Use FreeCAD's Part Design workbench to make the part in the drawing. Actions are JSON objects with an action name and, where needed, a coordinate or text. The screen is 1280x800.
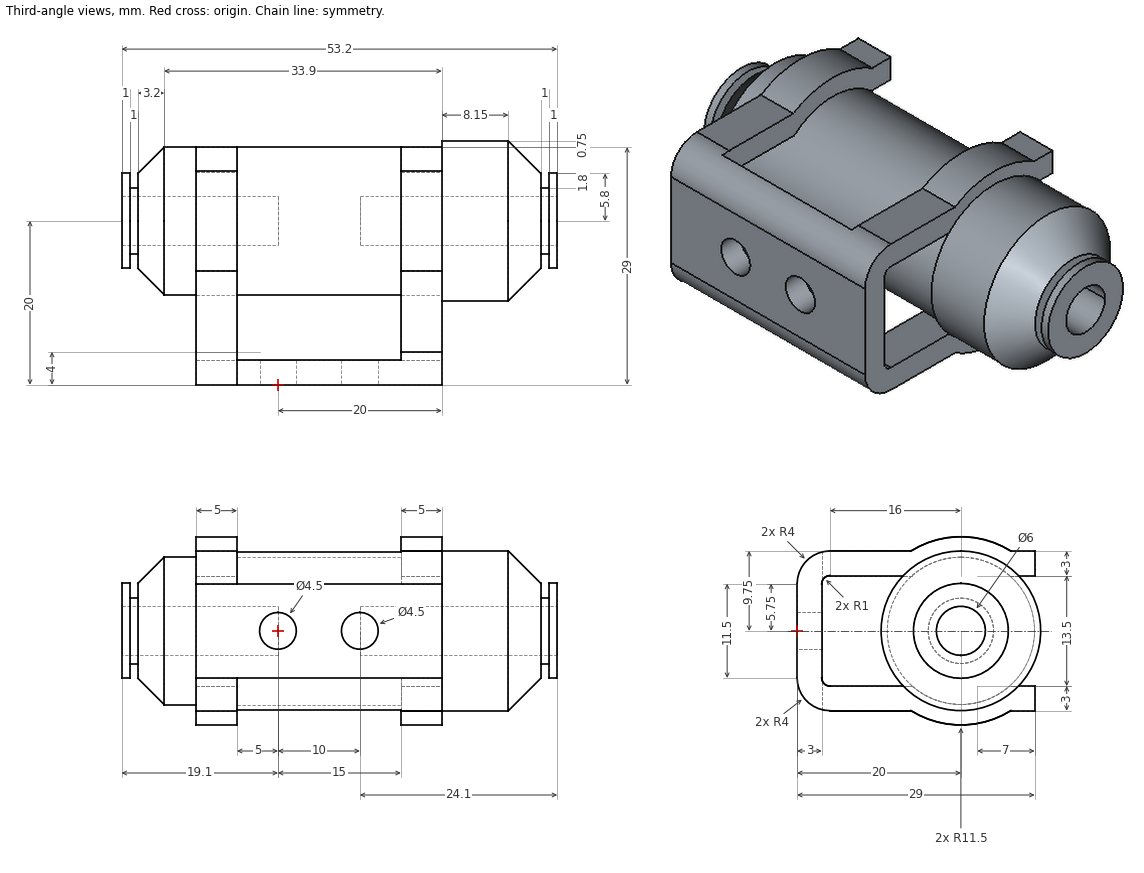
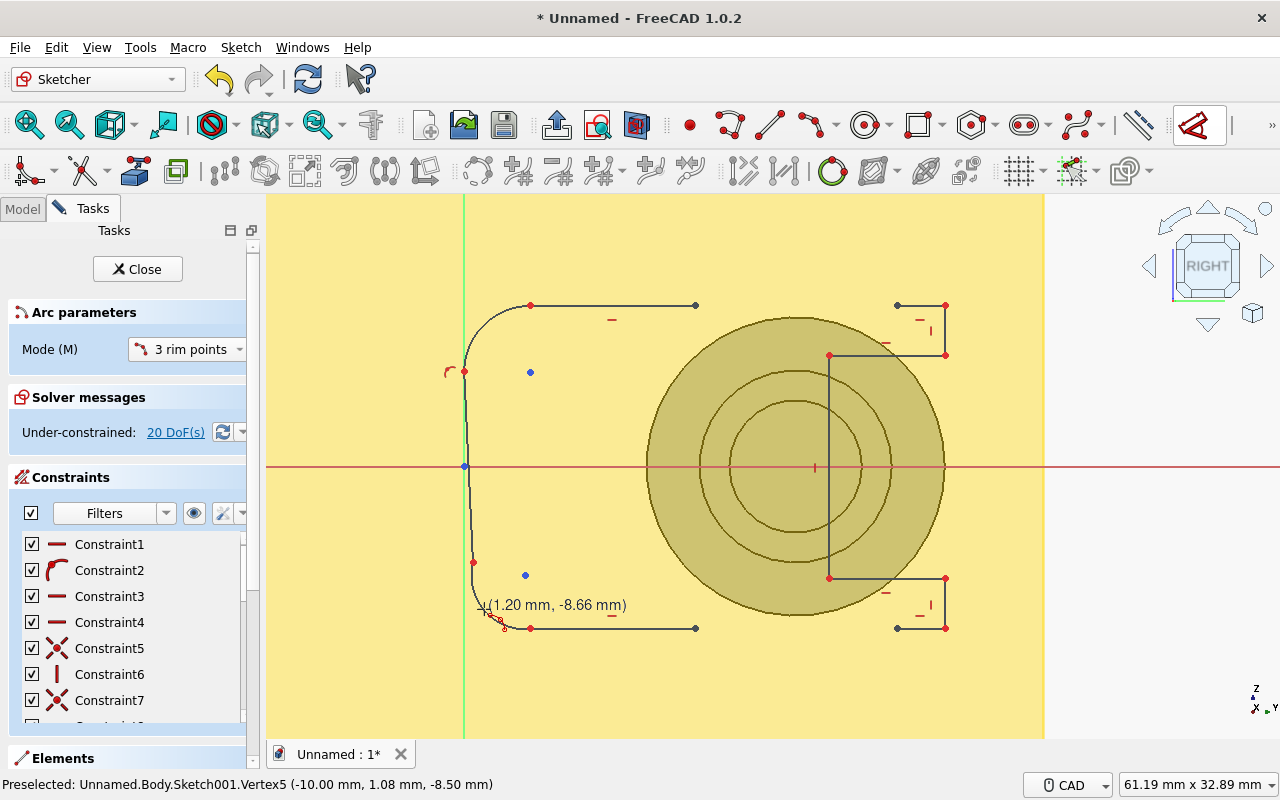
{"action": "left_click", "coordinate": [695, 629]}
{"action": "left_click", "coordinate": [897, 629]}
{"action": "left_click", "coordinate": [796, 657]}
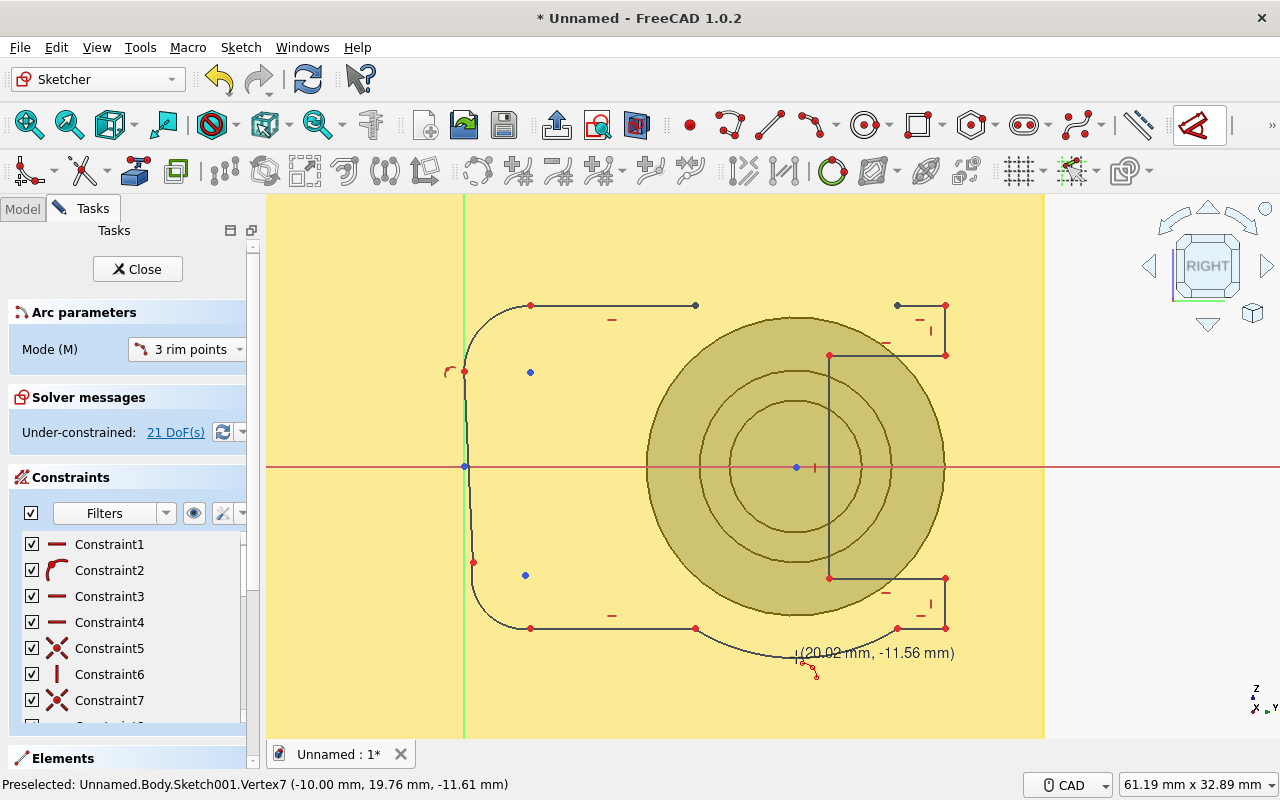
{"action": "left_click", "coordinate": [897, 306]}
{"action": "left_click", "coordinate": [695, 306]}
{"action": "left_click", "coordinate": [796, 276]}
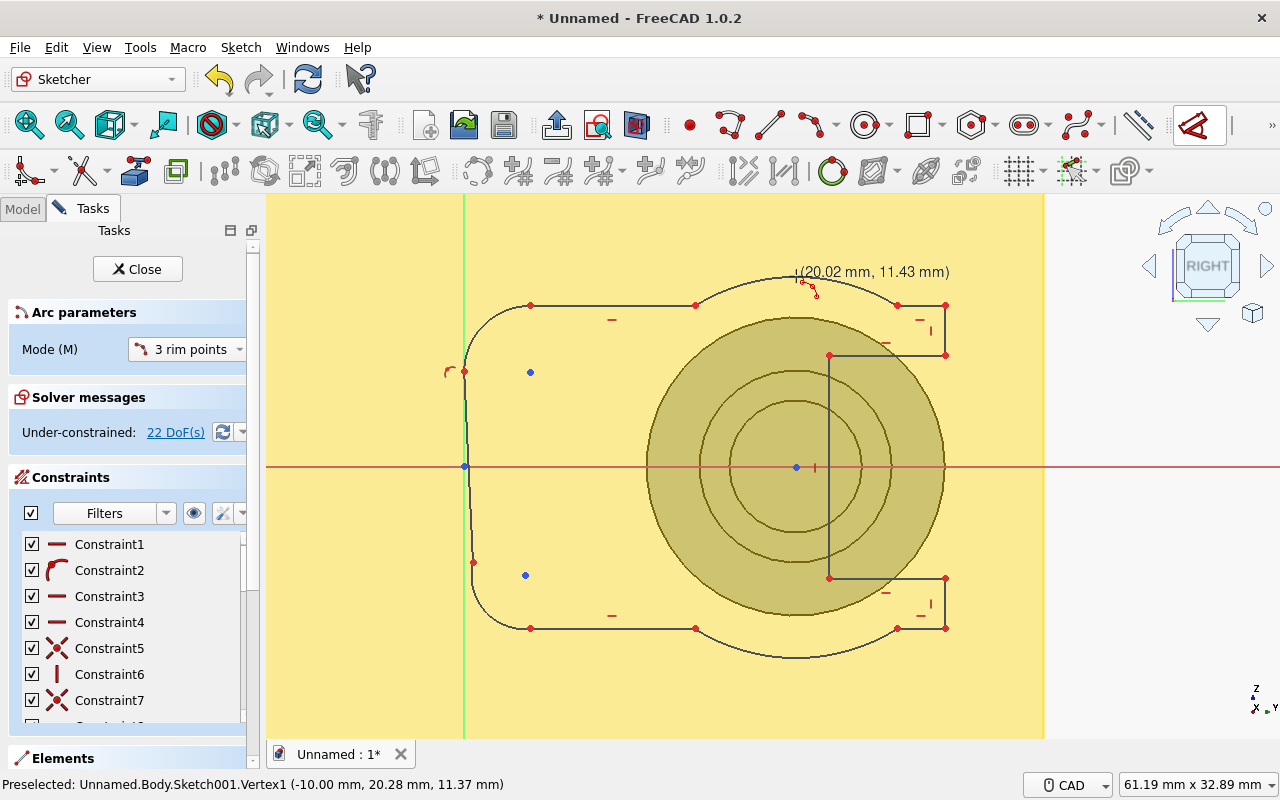
{"action": "left_click", "coordinate": [770, 126]}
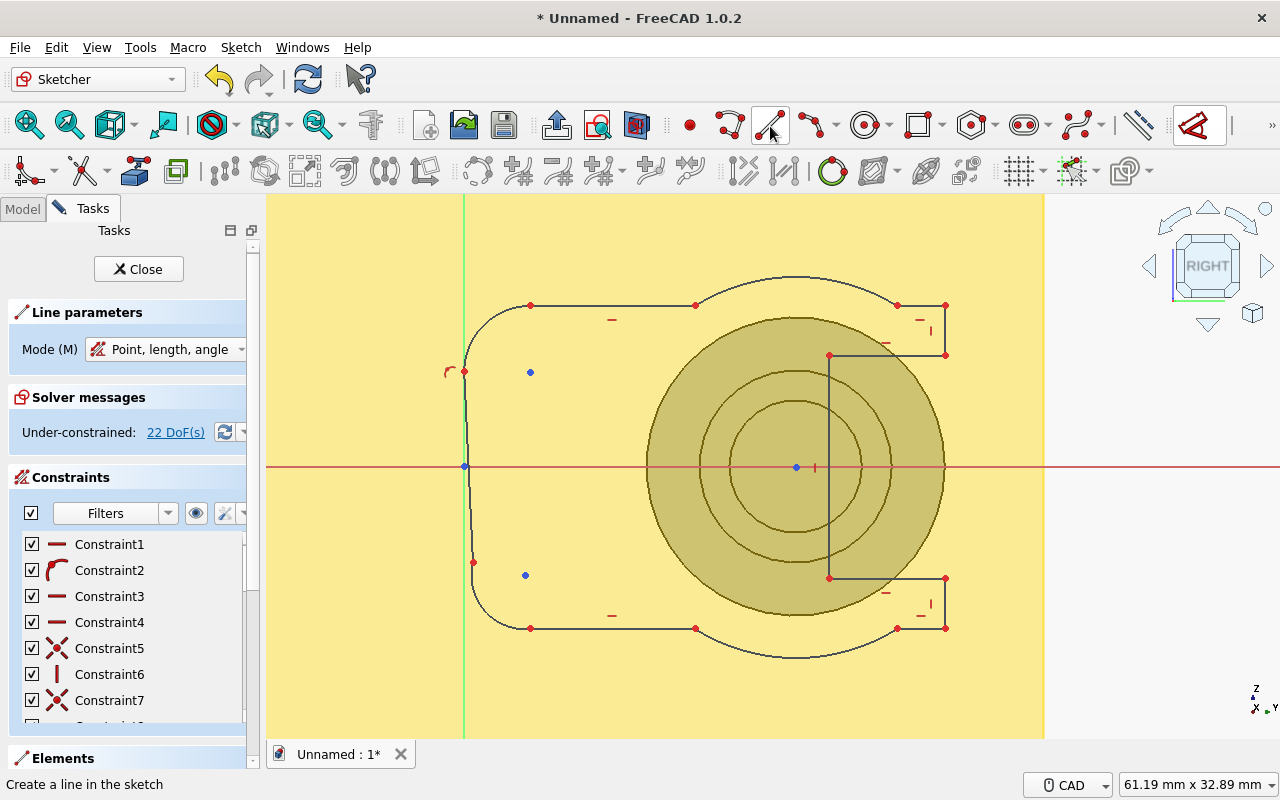
{"action": "left_click", "coordinate": [514, 562]}
{"action": "left_click", "coordinate": [514, 371]}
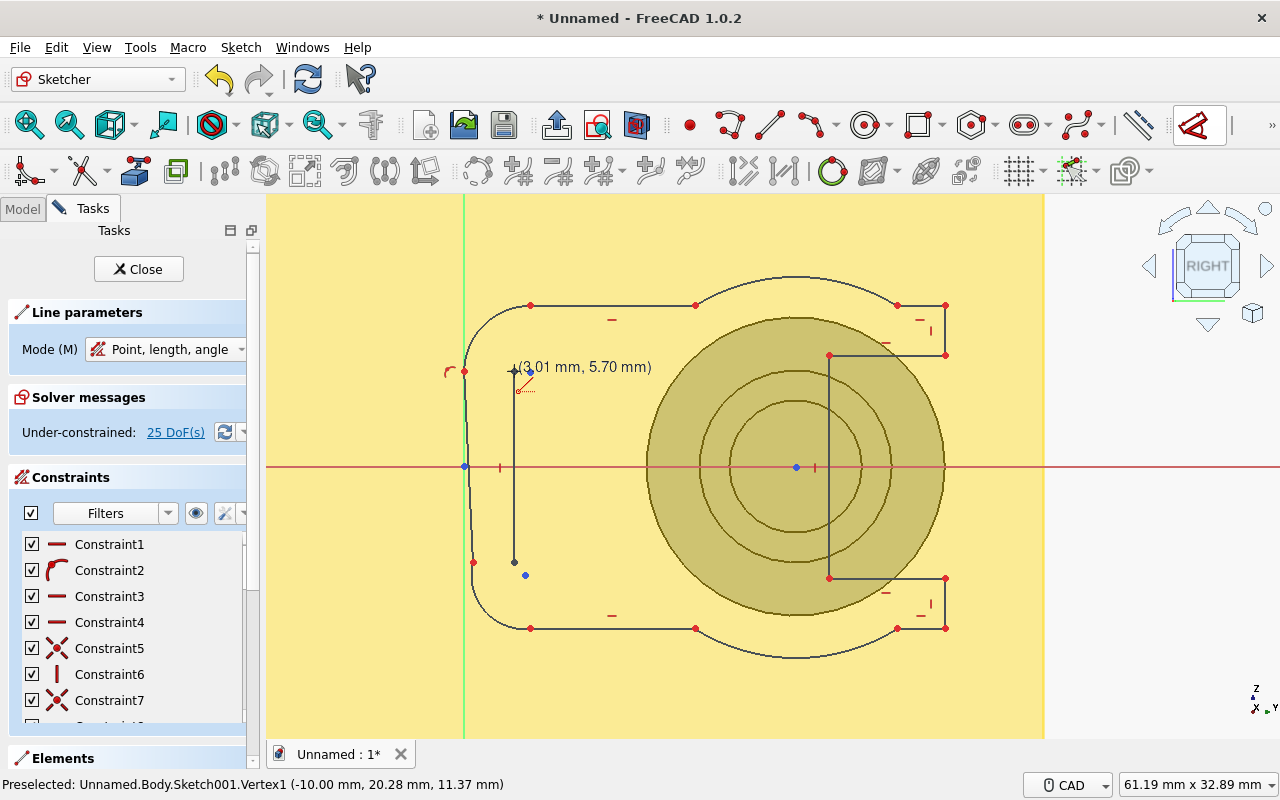
{"action": "left_click", "coordinate": [730, 126]}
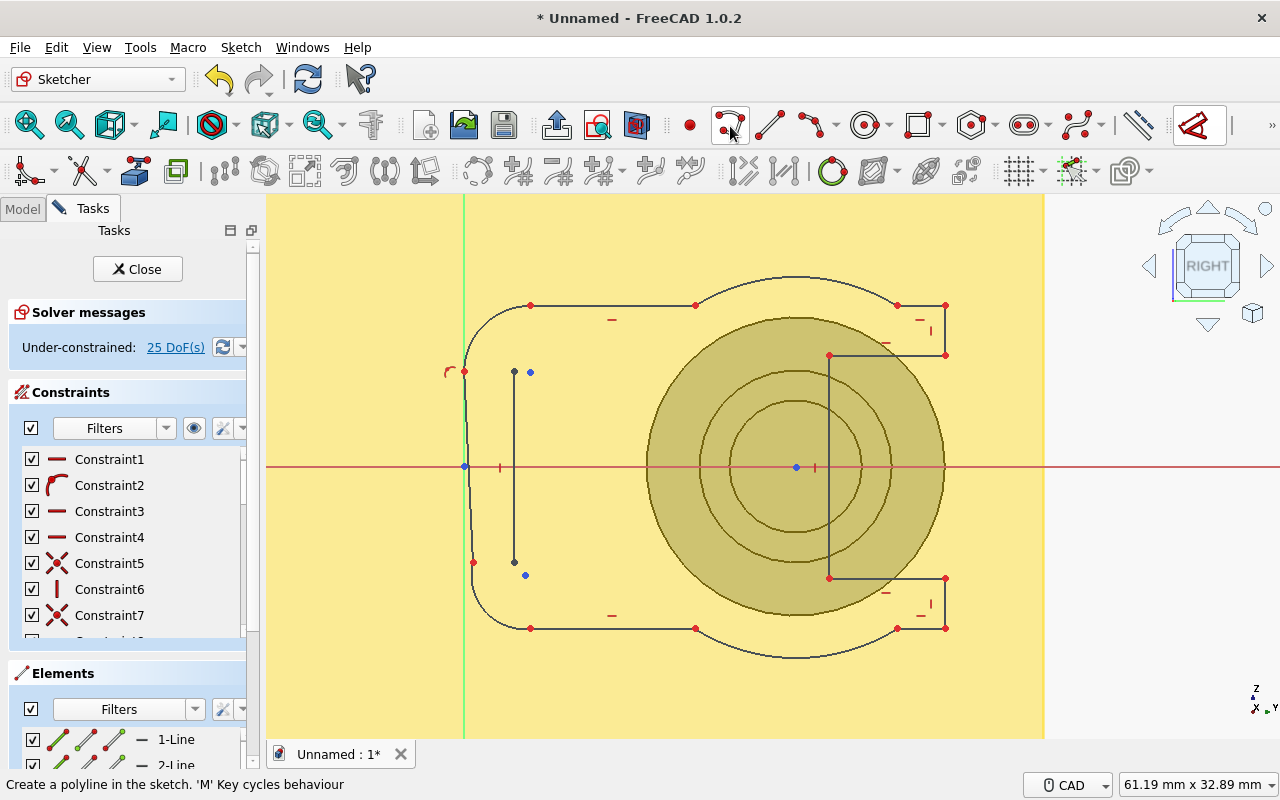
{"action": "left_click", "coordinate": [530, 355]}
{"action": "left_click", "coordinate": [796, 355]}
{"action": "left_click", "coordinate": [796, 578]}
{"action": "left_click", "coordinate": [530, 578]}
{"action": "right_click", "coordinate": [530, 578]}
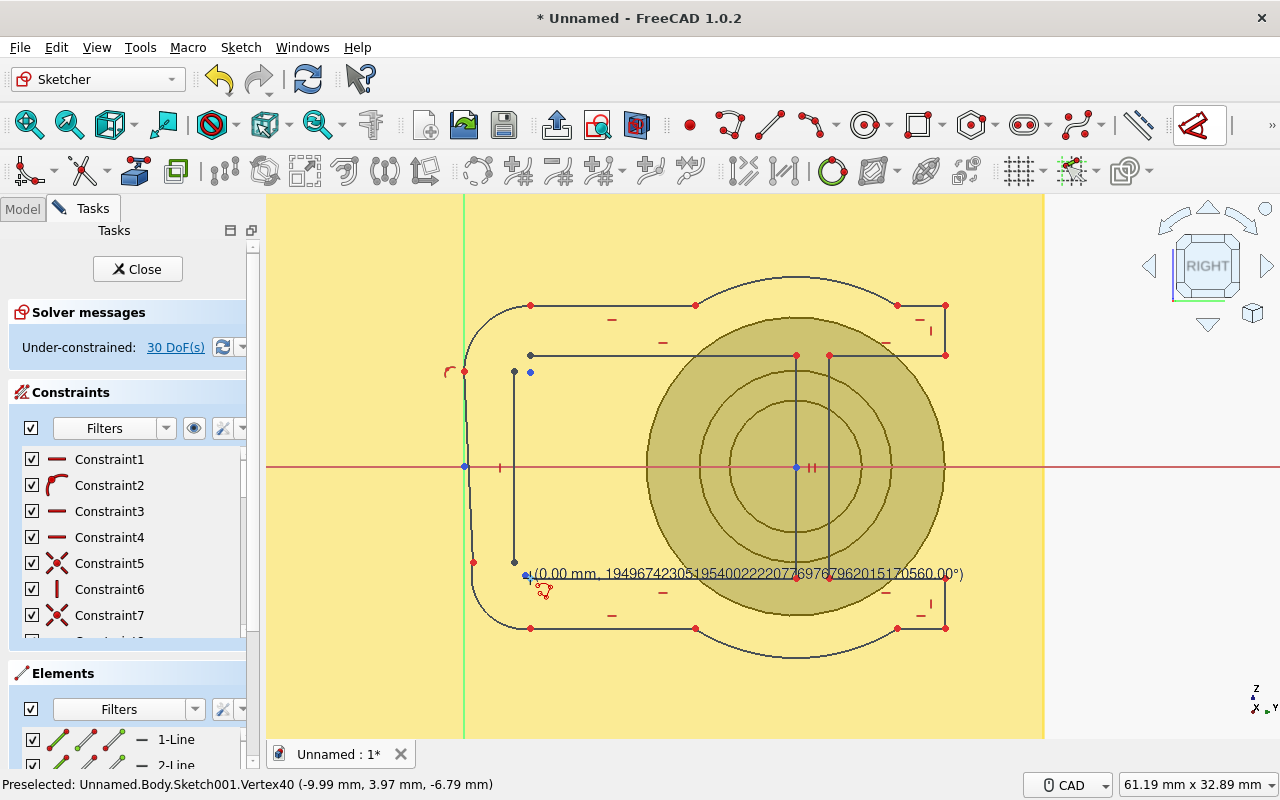
{"action": "left_click", "coordinate": [812, 126]}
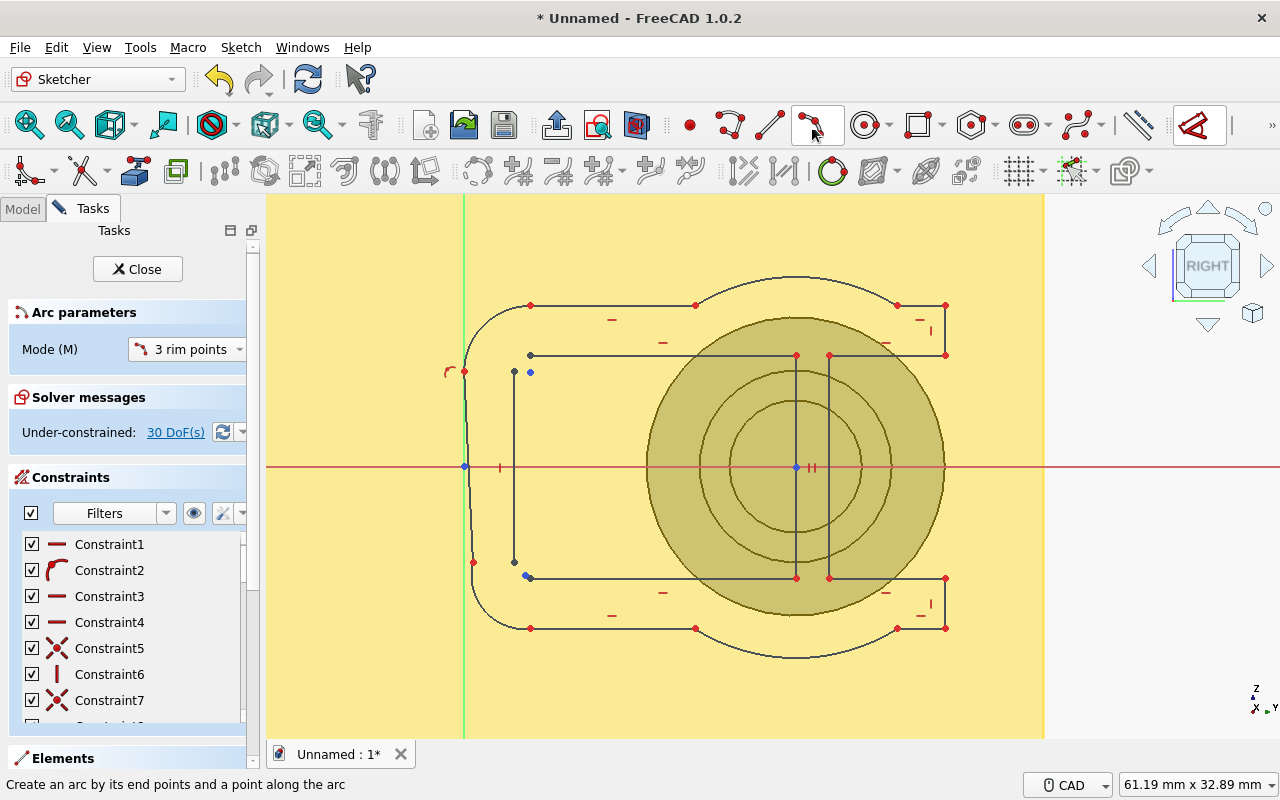
{"action": "left_click", "coordinate": [514, 372]}
{"action": "left_click", "coordinate": [530, 356]}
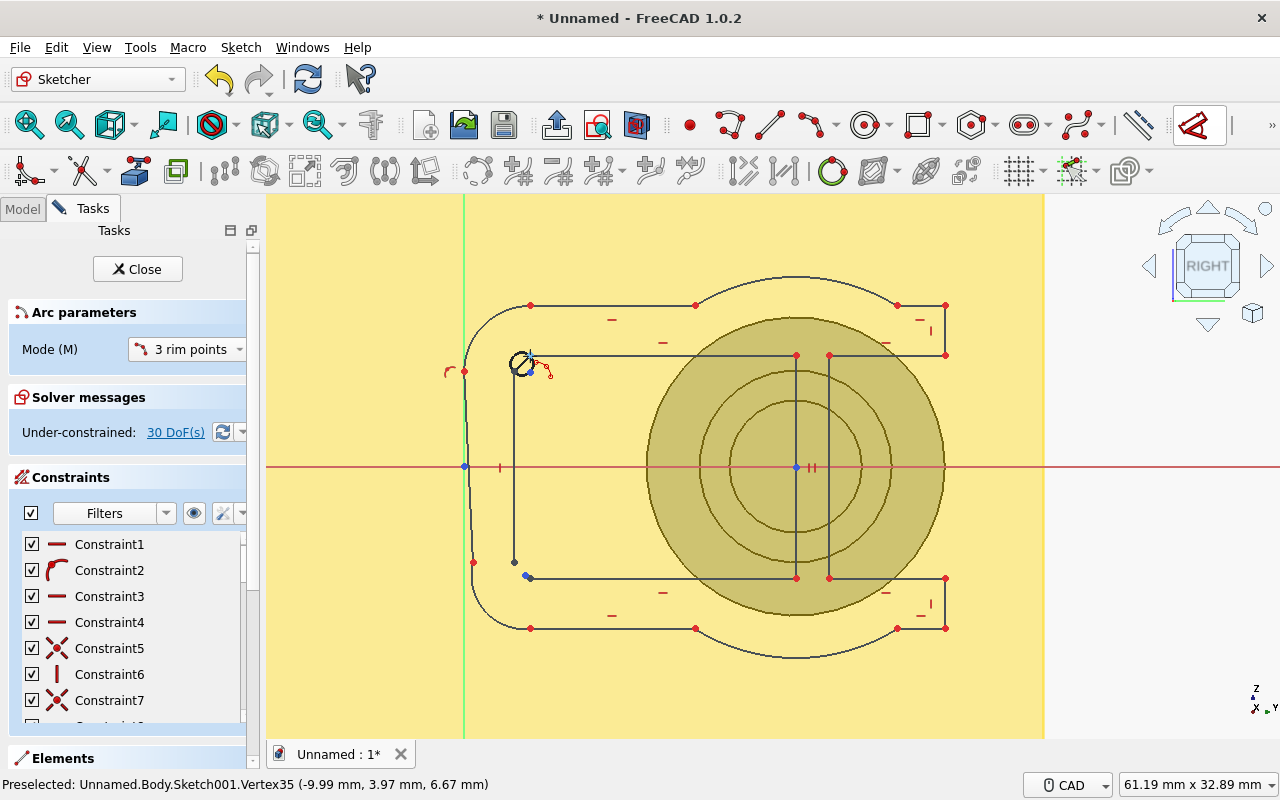
{"action": "scroll", "coordinate": [519, 359], "scroll_direction": "up", "scroll_amount": 6}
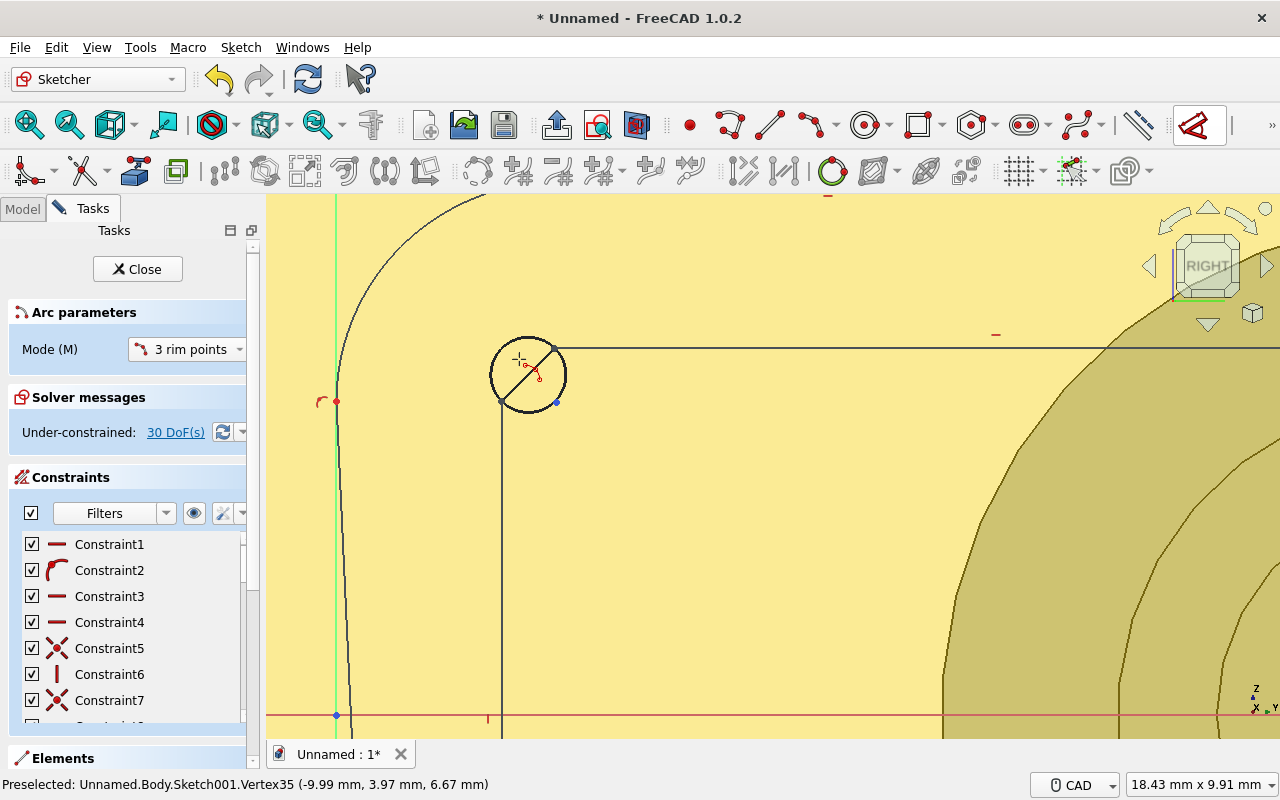
{"action": "left_click", "coordinate": [518, 360]}